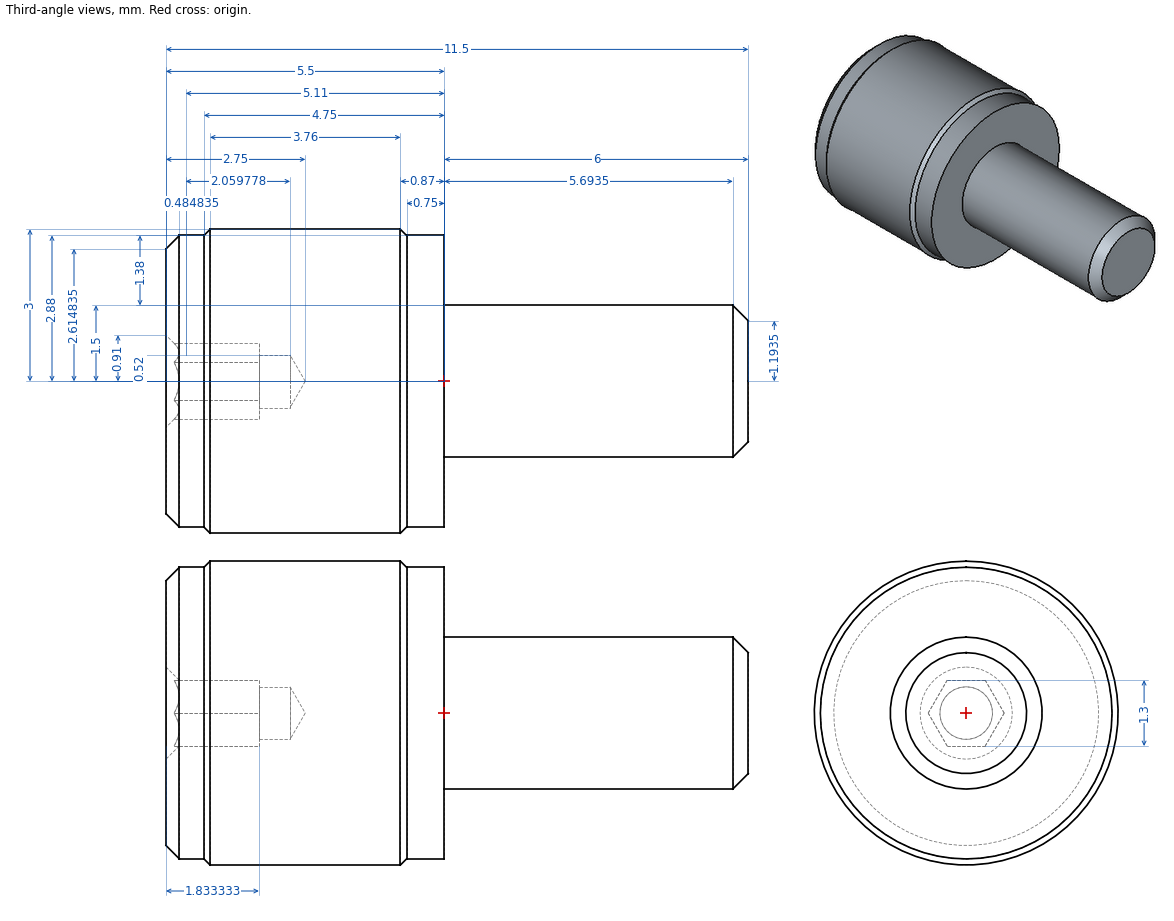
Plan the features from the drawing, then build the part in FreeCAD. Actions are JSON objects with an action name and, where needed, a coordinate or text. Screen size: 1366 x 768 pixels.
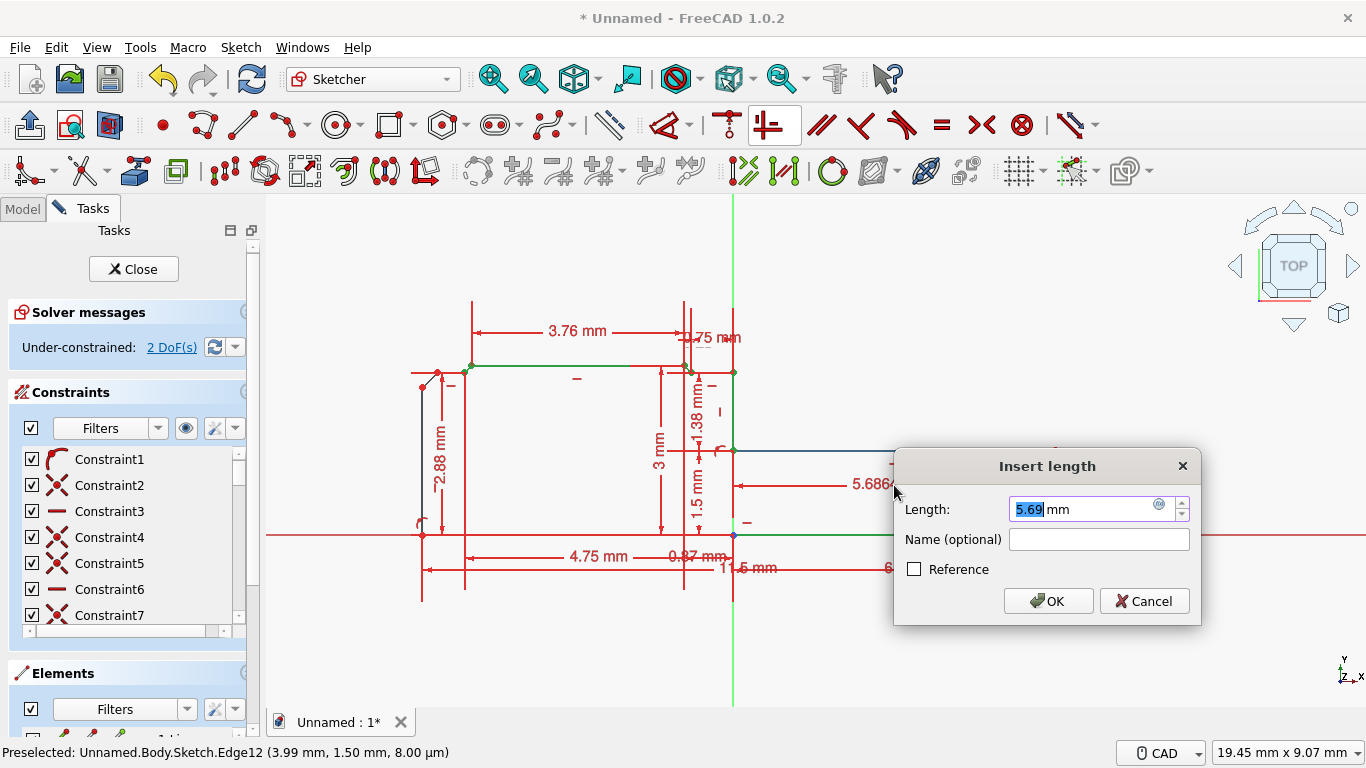
{"action": "type", "text": "5.6935"}
{"action": "key", "text": "Return"}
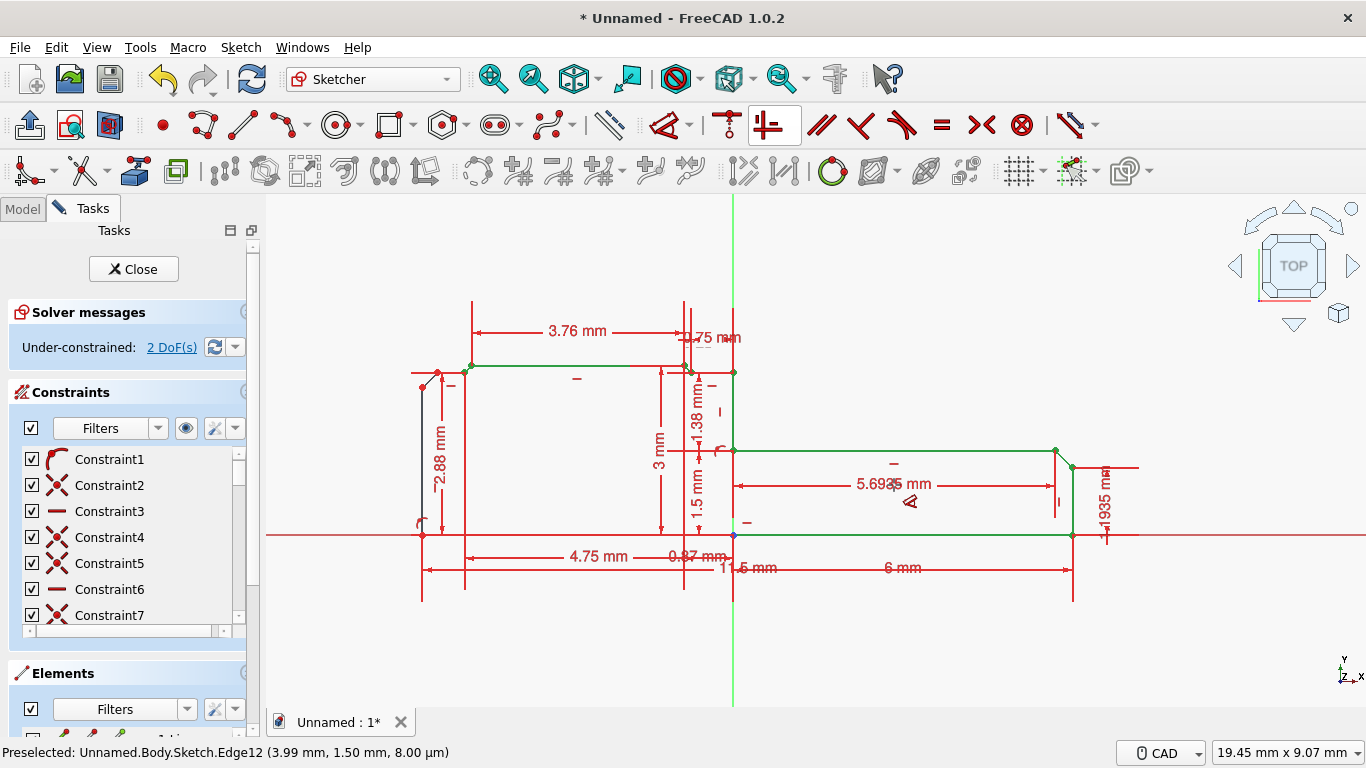
{"action": "scroll", "coordinate": [454, 373], "scroll_direction": "up", "scroll_amount": 2}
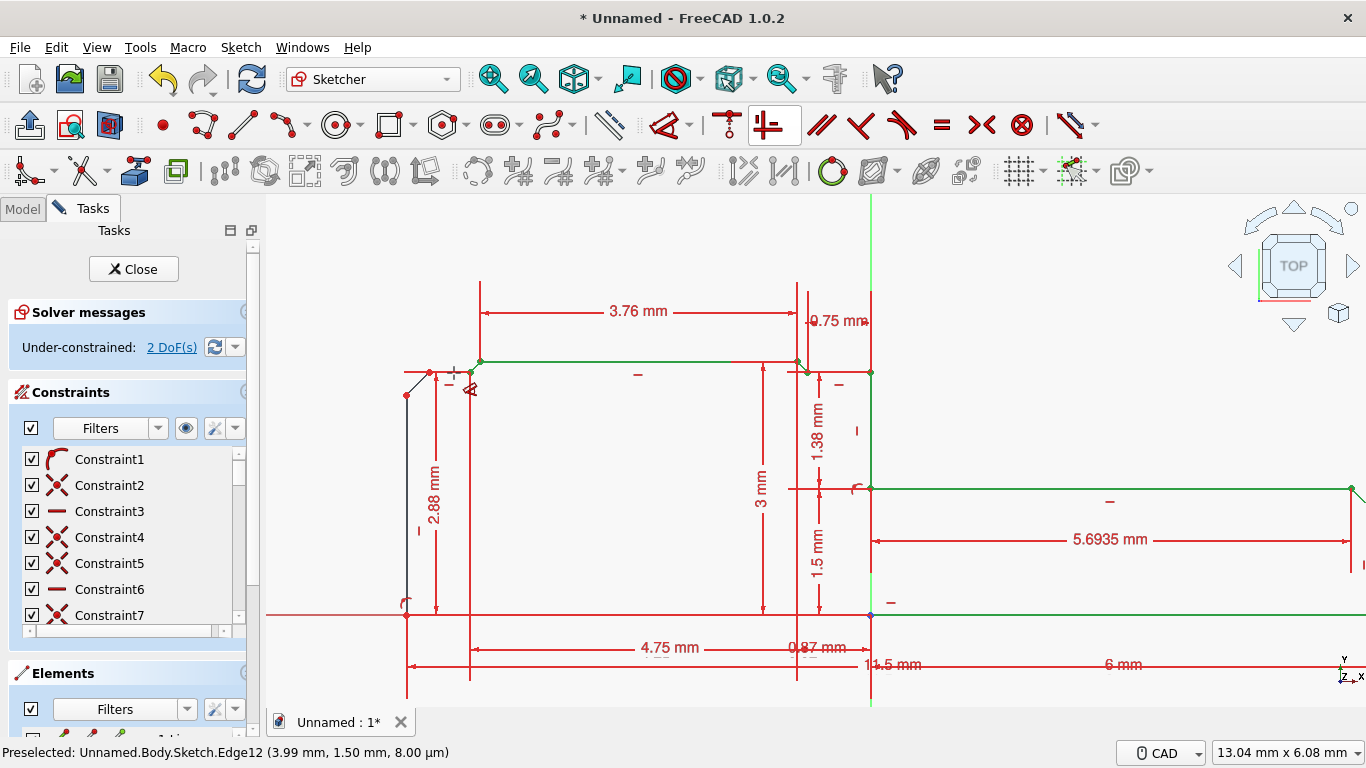
{"action": "left_click", "coordinate": [454, 372]}
{"action": "left_click", "coordinate": [450, 338]}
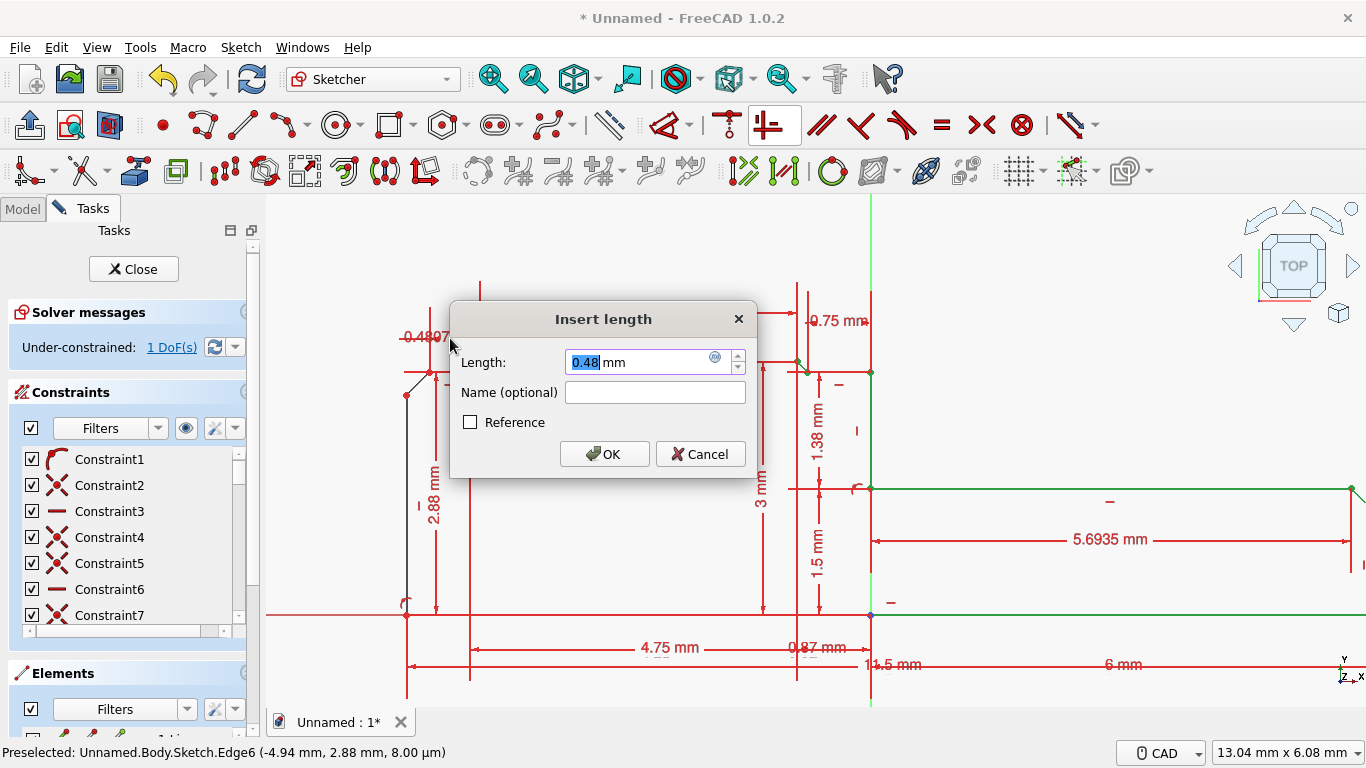
{"action": "type", "text": "0.484835"}
{"action": "key", "text": "Return"}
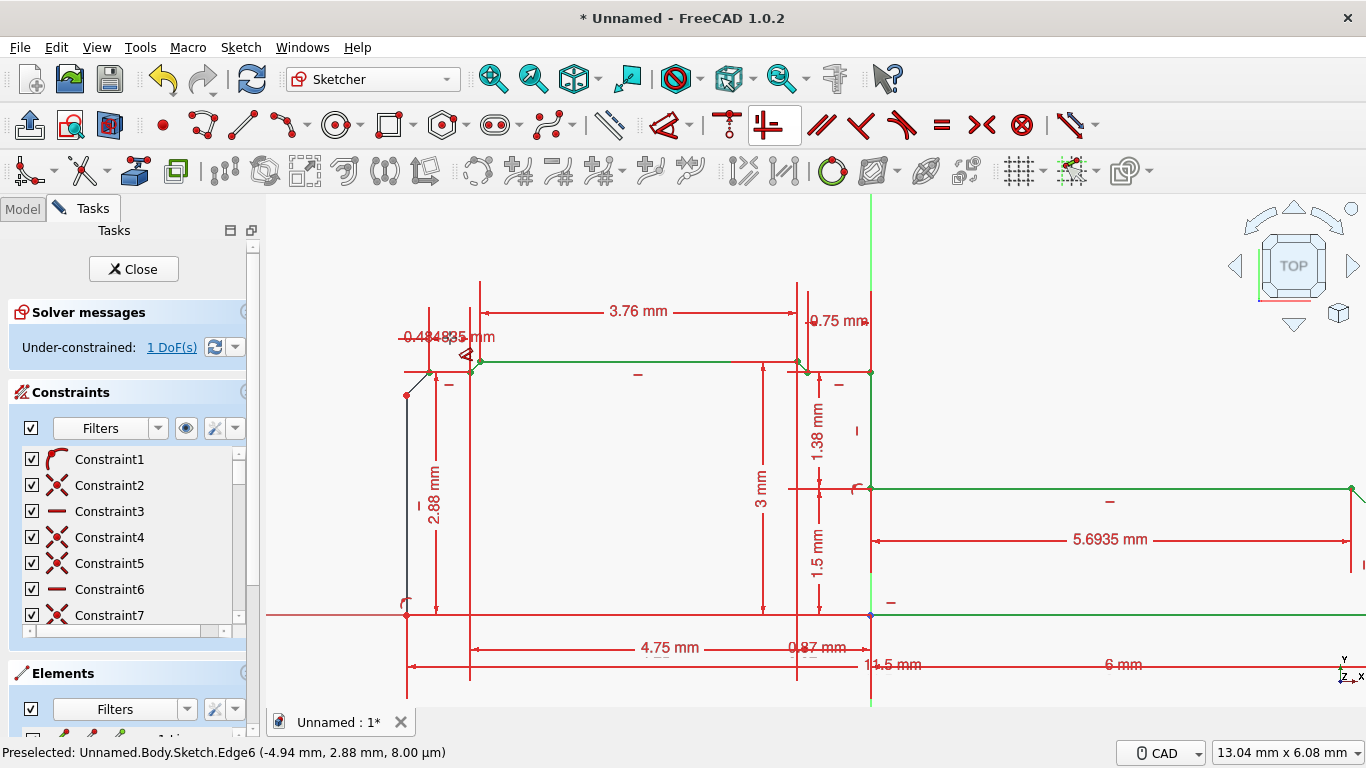
{"action": "left_click", "coordinate": [407, 461]}
{"action": "left_click", "coordinate": [373, 455]}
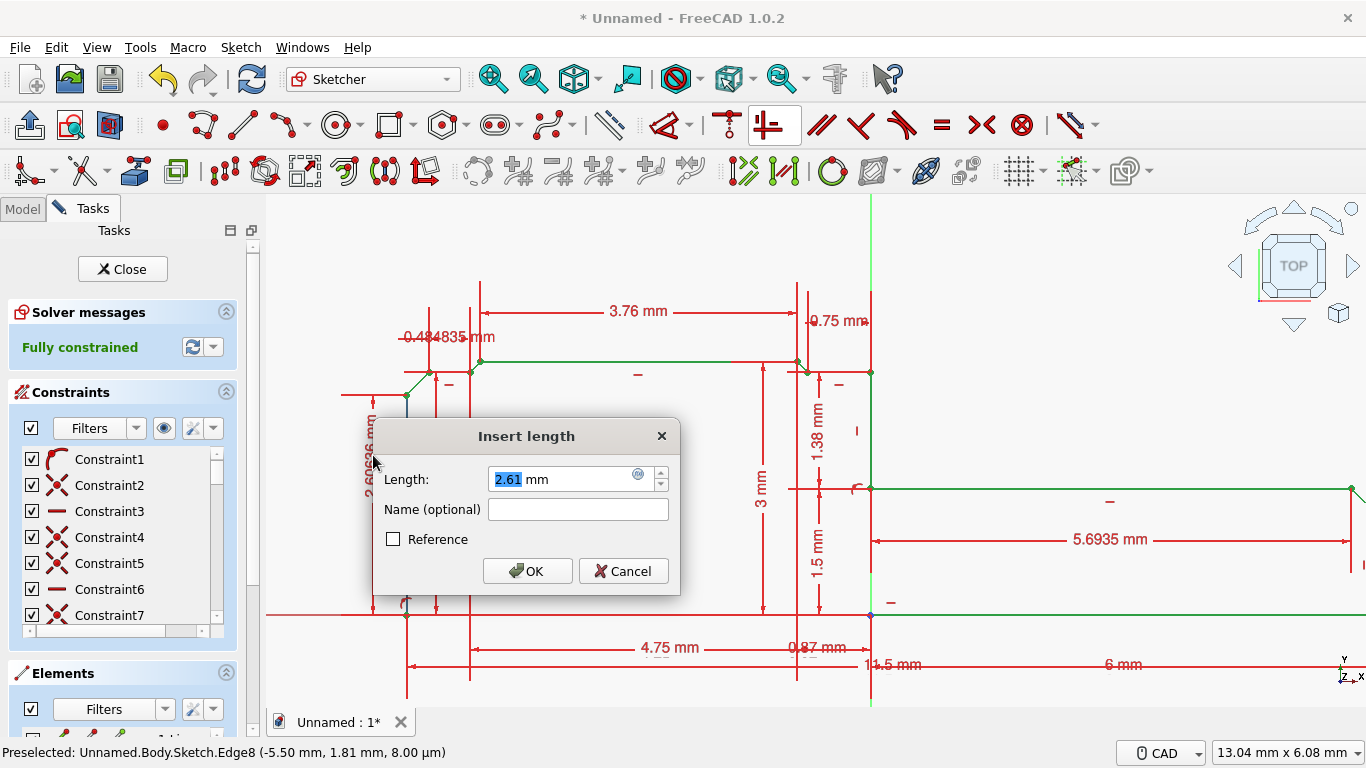
{"action": "type", "text": "2.614835"}
{"action": "key", "text": "Return"}
{"action": "key", "text": "Escape"}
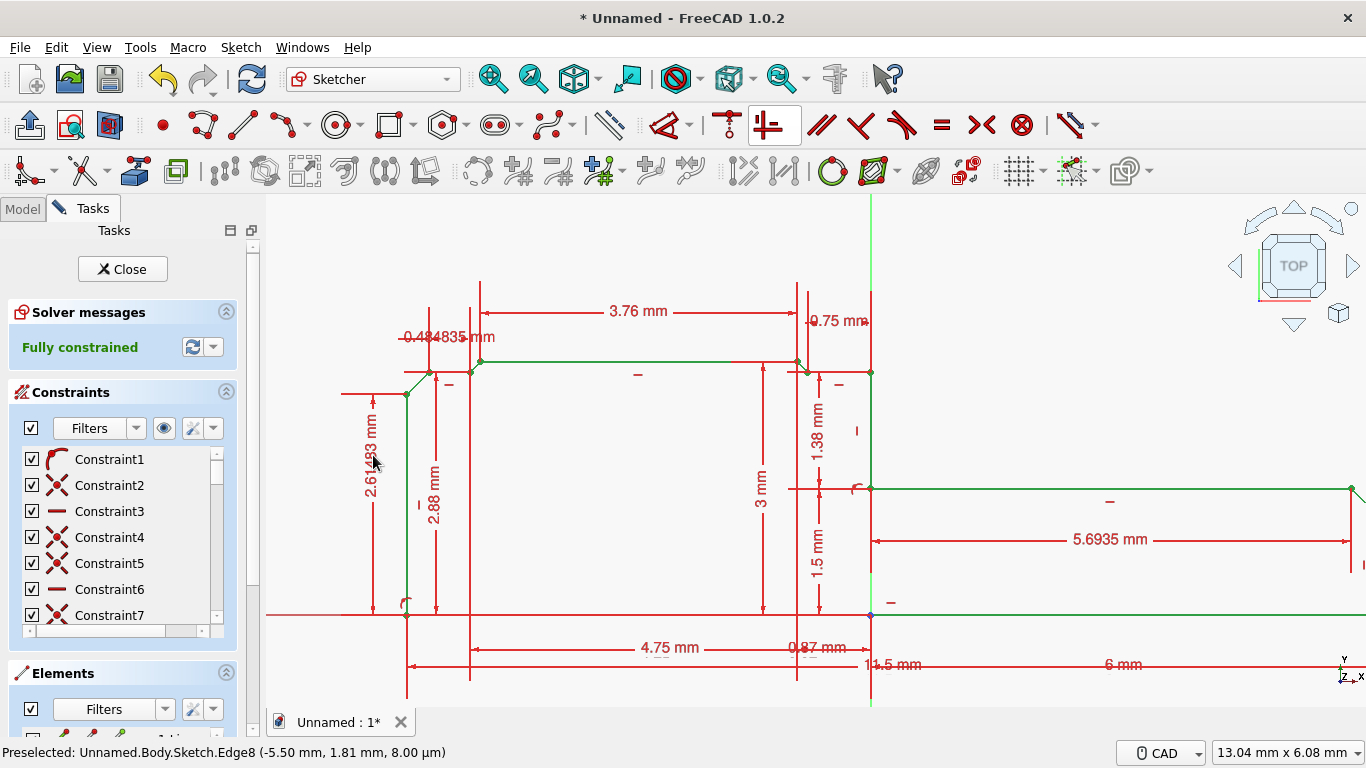
{"action": "left_click", "coordinate": [123, 269]}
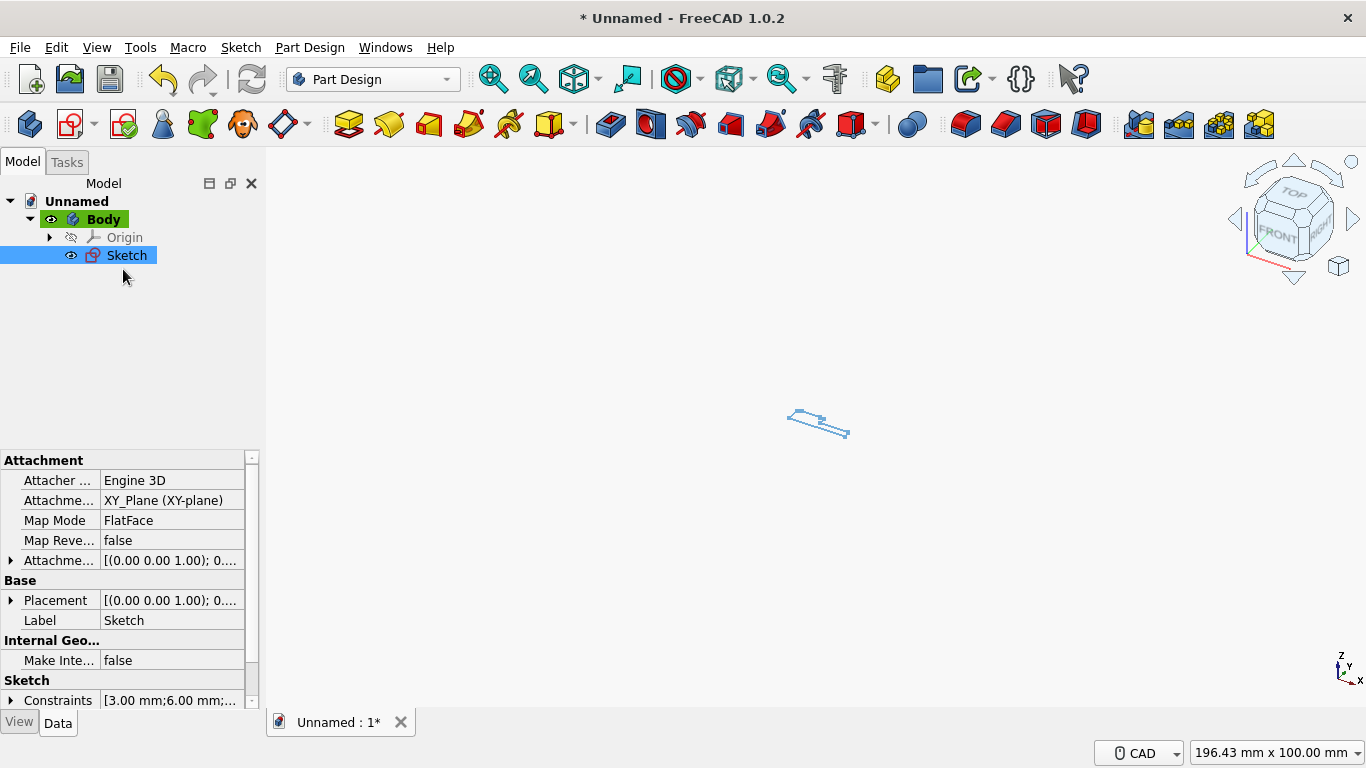
{"action": "left_click", "coordinate": [390, 124]}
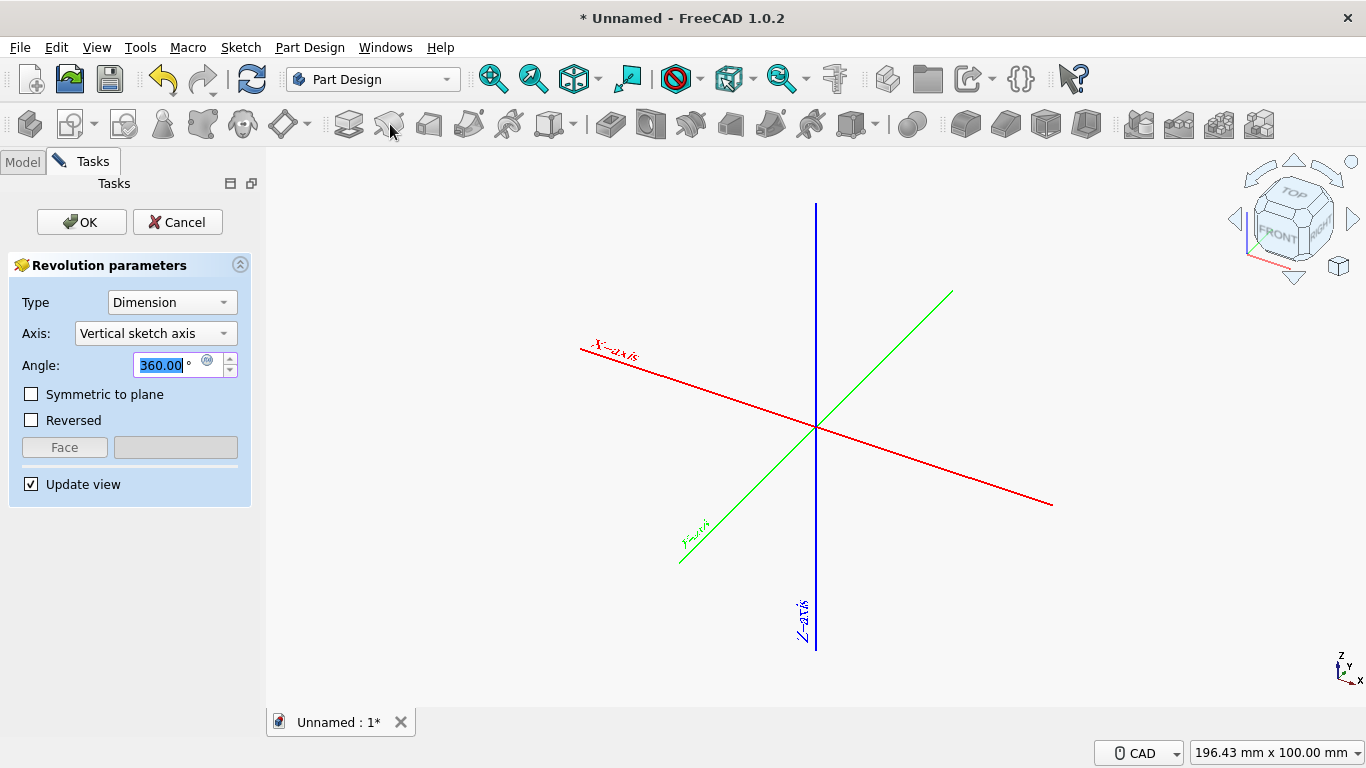
{"action": "left_click", "coordinate": [156, 334]}